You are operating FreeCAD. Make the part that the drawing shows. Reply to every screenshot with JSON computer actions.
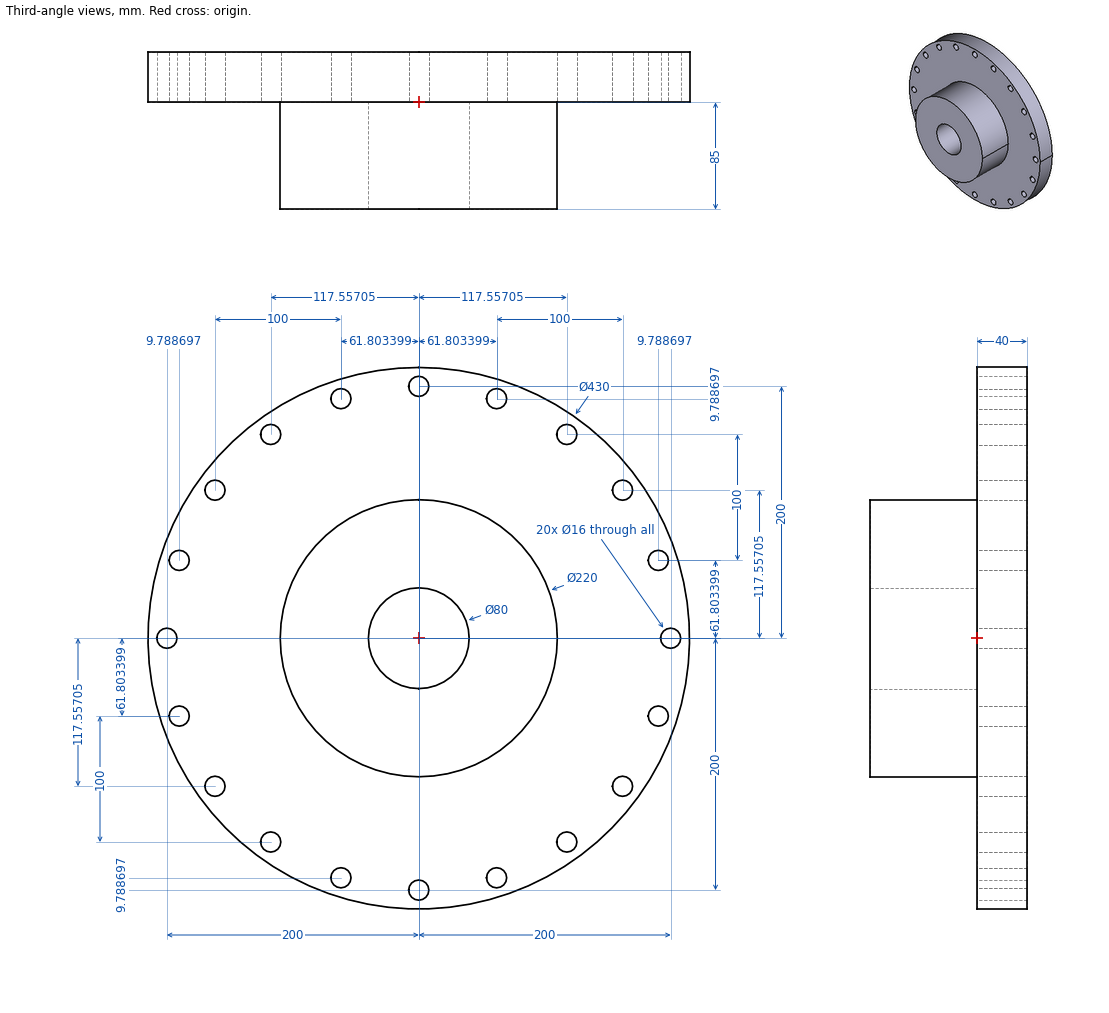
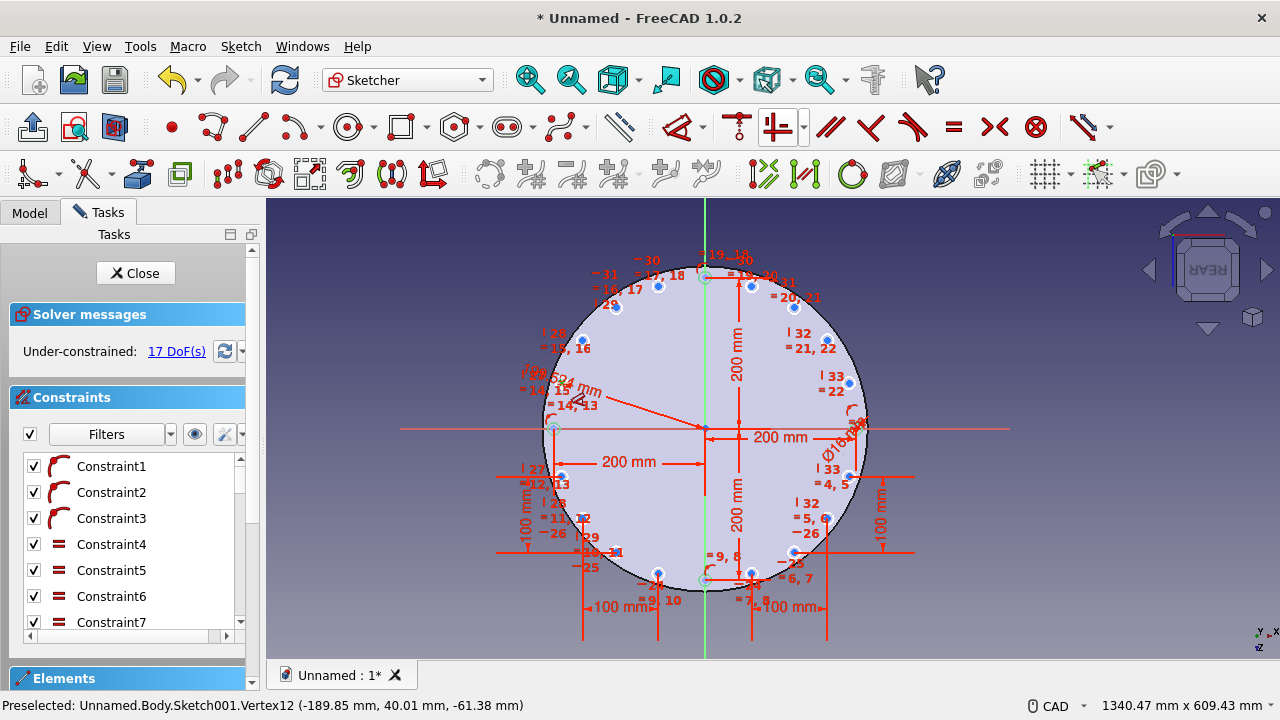
{"action": "left_click", "coordinate": [616, 308]}
{"action": "left_click", "coordinate": [528, 345]}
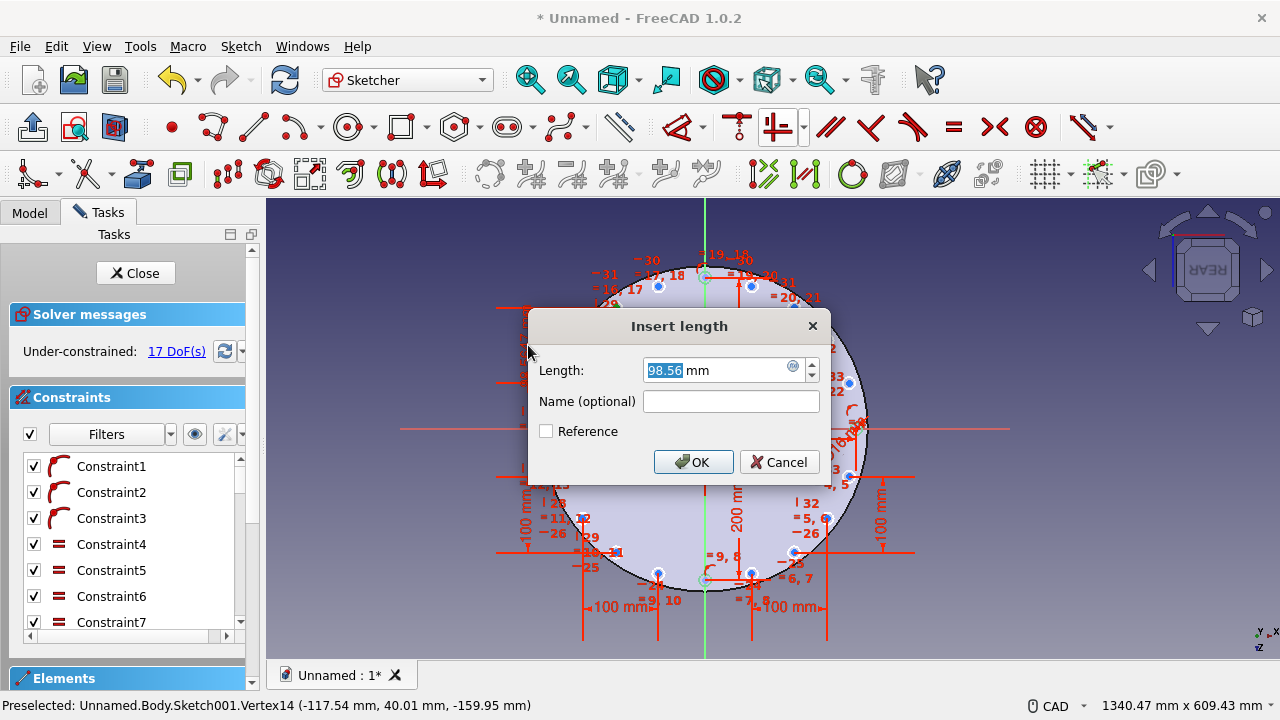
{"action": "type", "text": "100"}
{"action": "key", "text": "Return"}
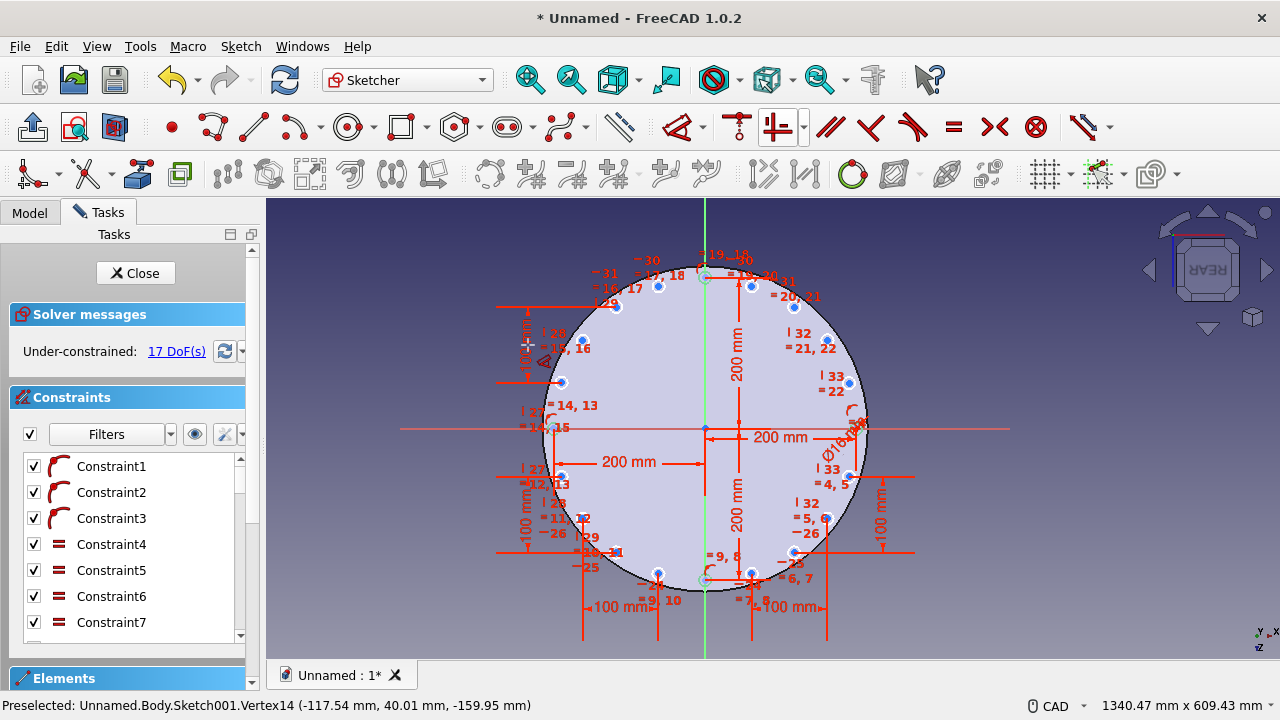
{"action": "left_click", "coordinate": [583, 341]}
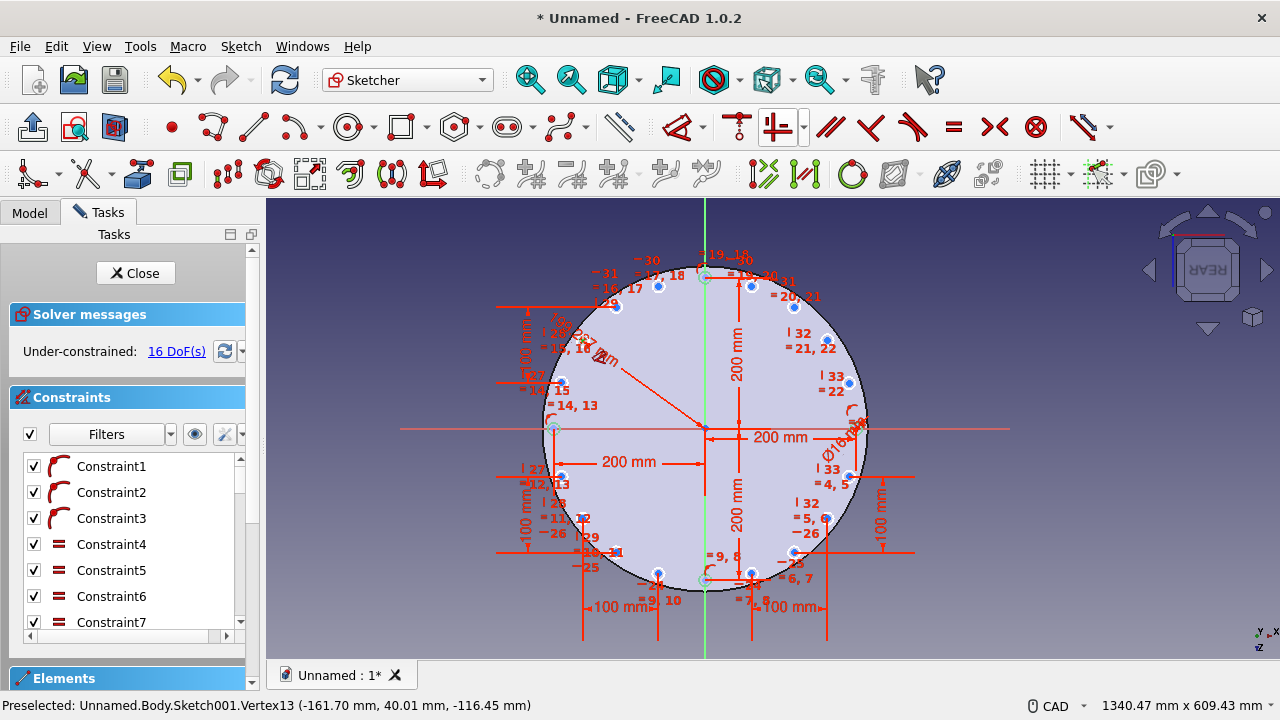
{"action": "left_click", "coordinate": [659, 286]}
{"action": "left_click", "coordinate": [621, 252]}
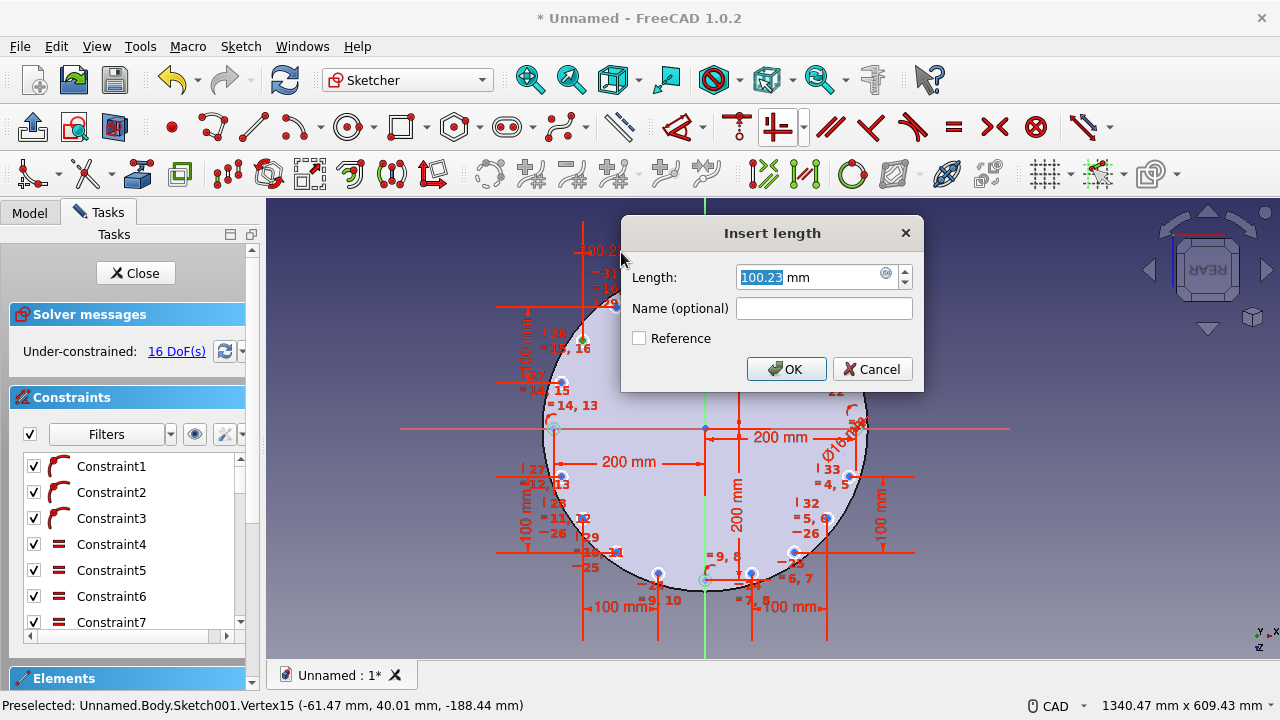
{"action": "type", "text": "100"}
{"action": "key", "text": "Return"}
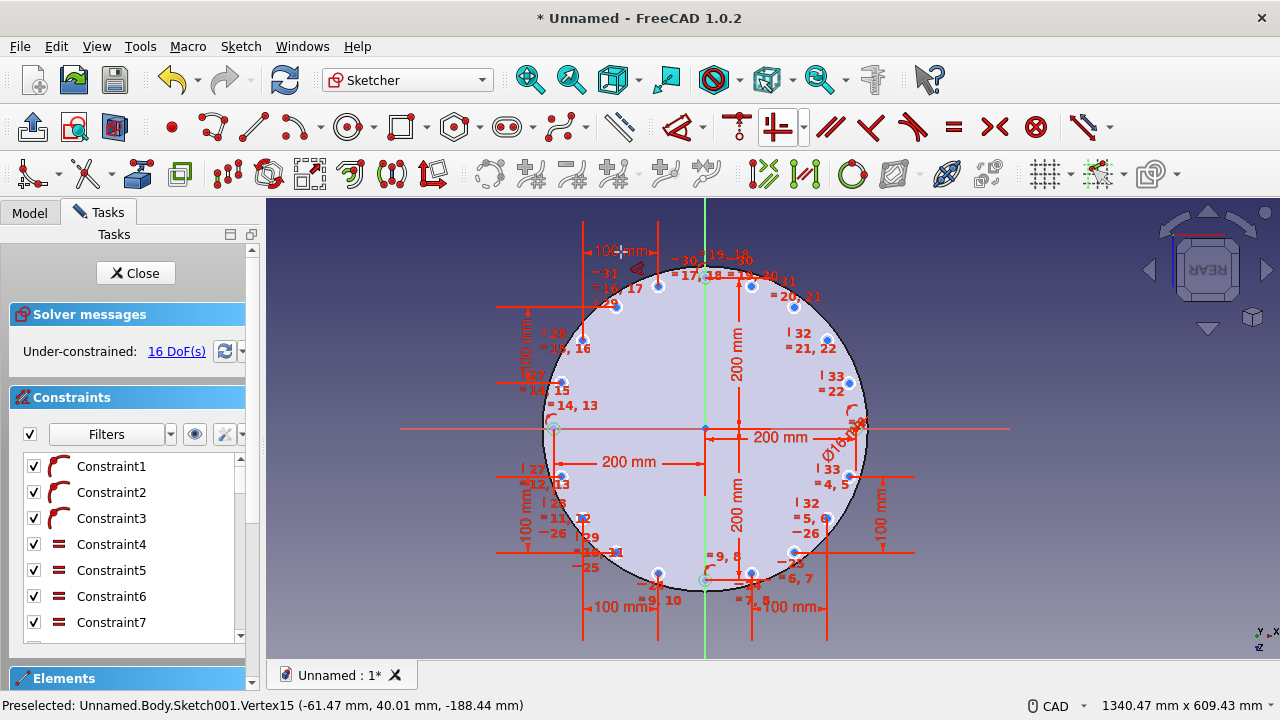
{"action": "left_click", "coordinate": [752, 286]}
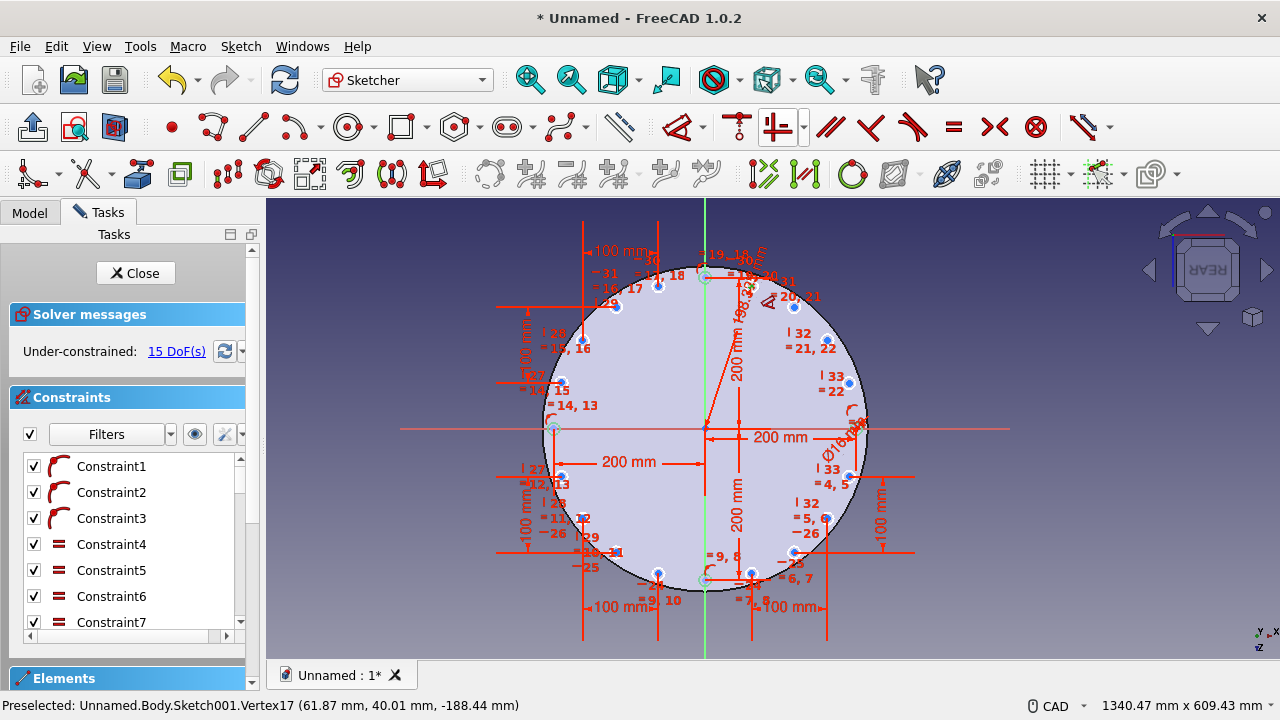
{"action": "left_click", "coordinate": [827, 340]}
{"action": "left_click", "coordinate": [790, 252]}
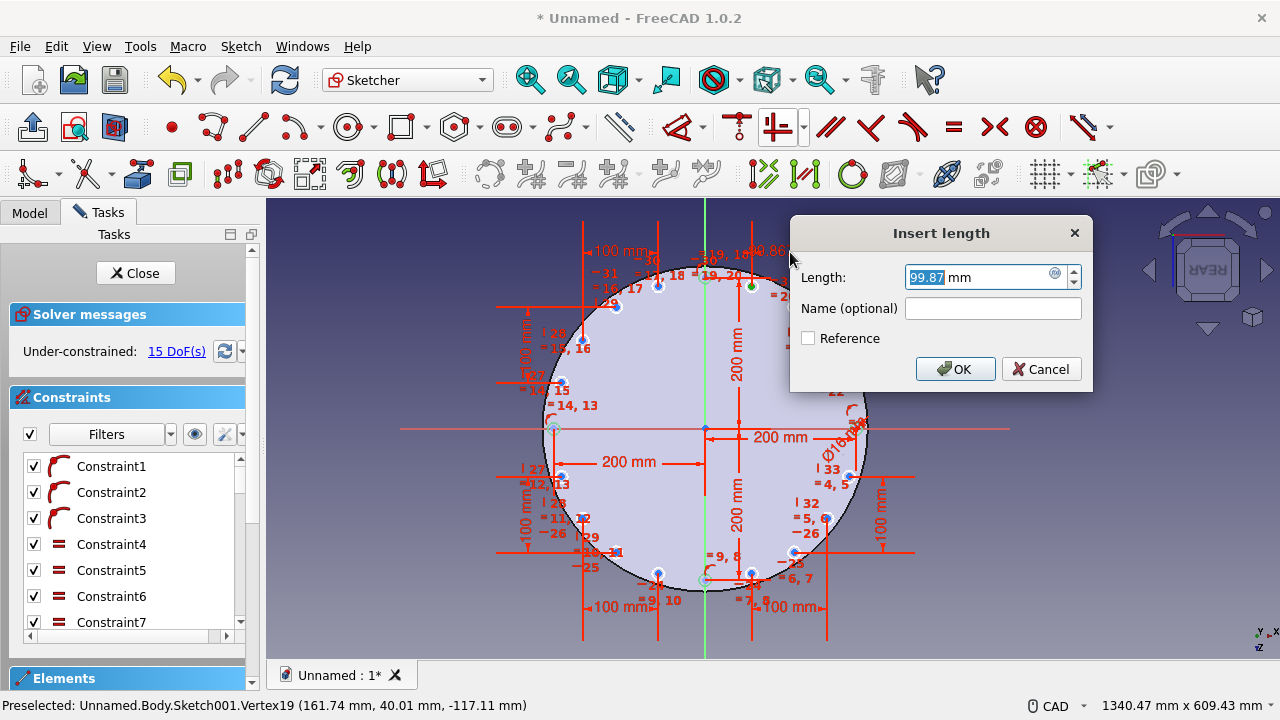
{"action": "type", "text": "100"}
{"action": "key", "text": "Return"}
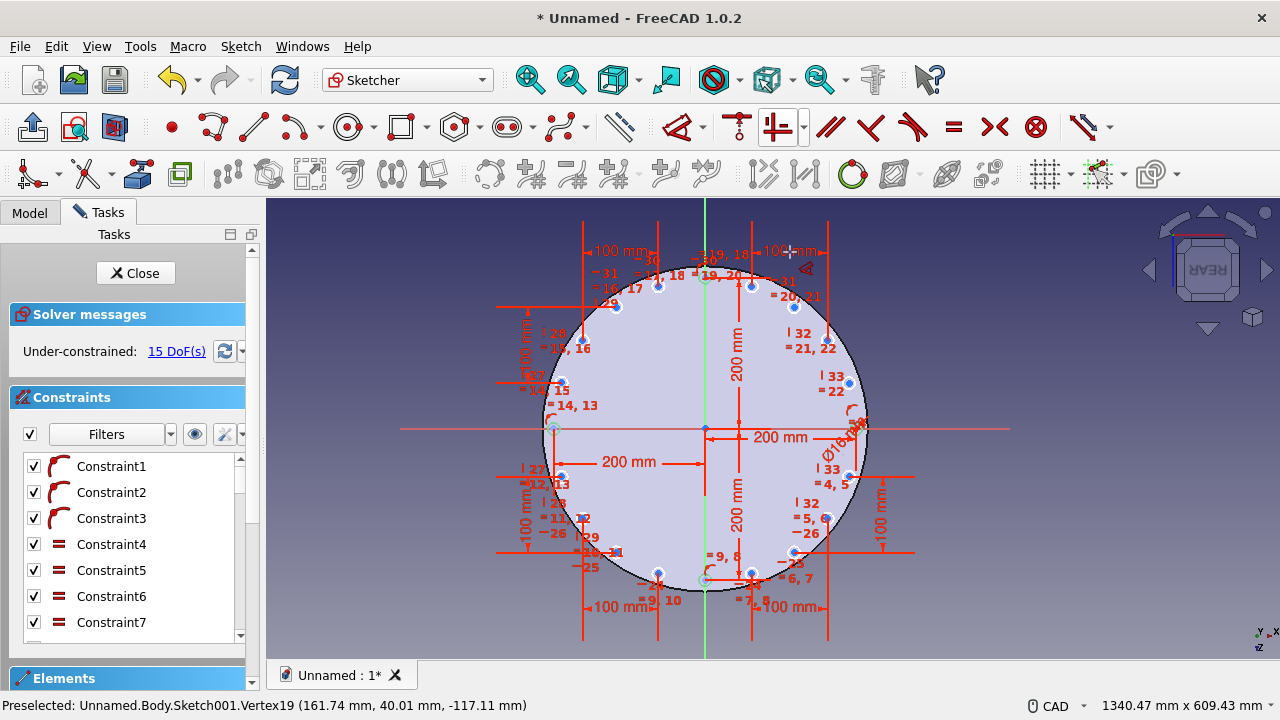
{"action": "left_click", "coordinate": [794, 307]}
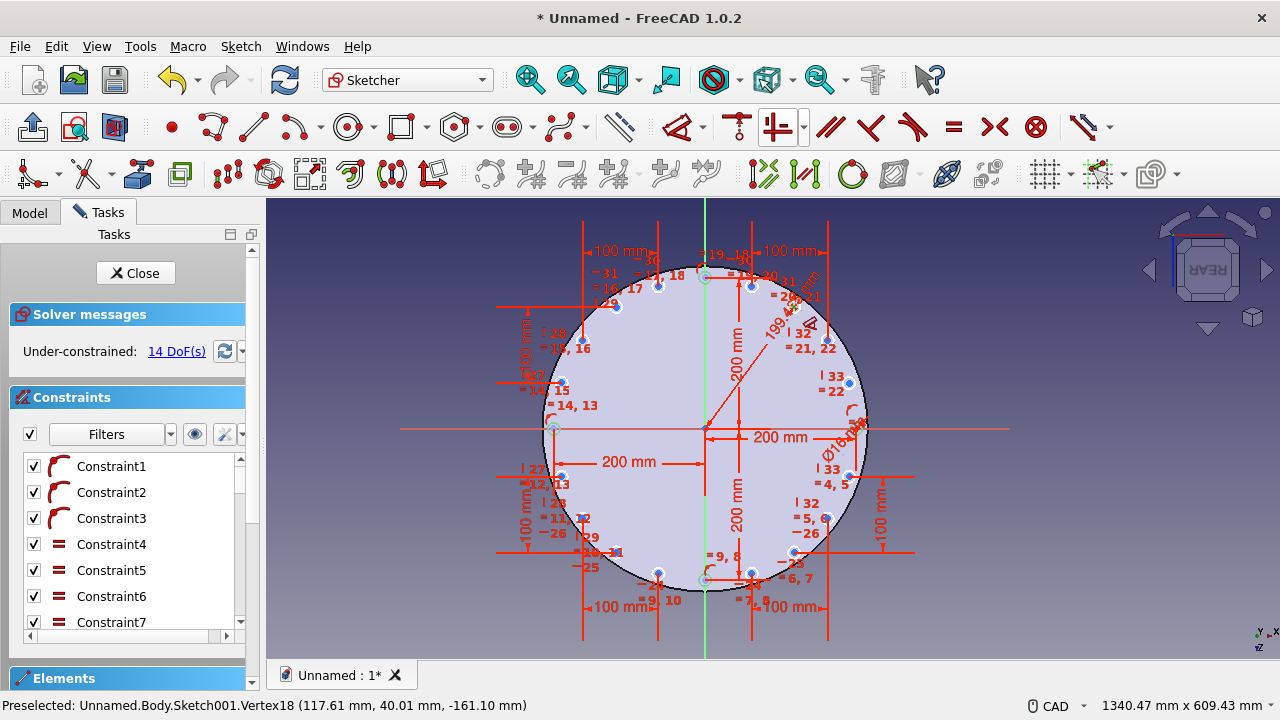
{"action": "left_click", "coordinate": [849, 383]}
{"action": "left_click", "coordinate": [883, 345]}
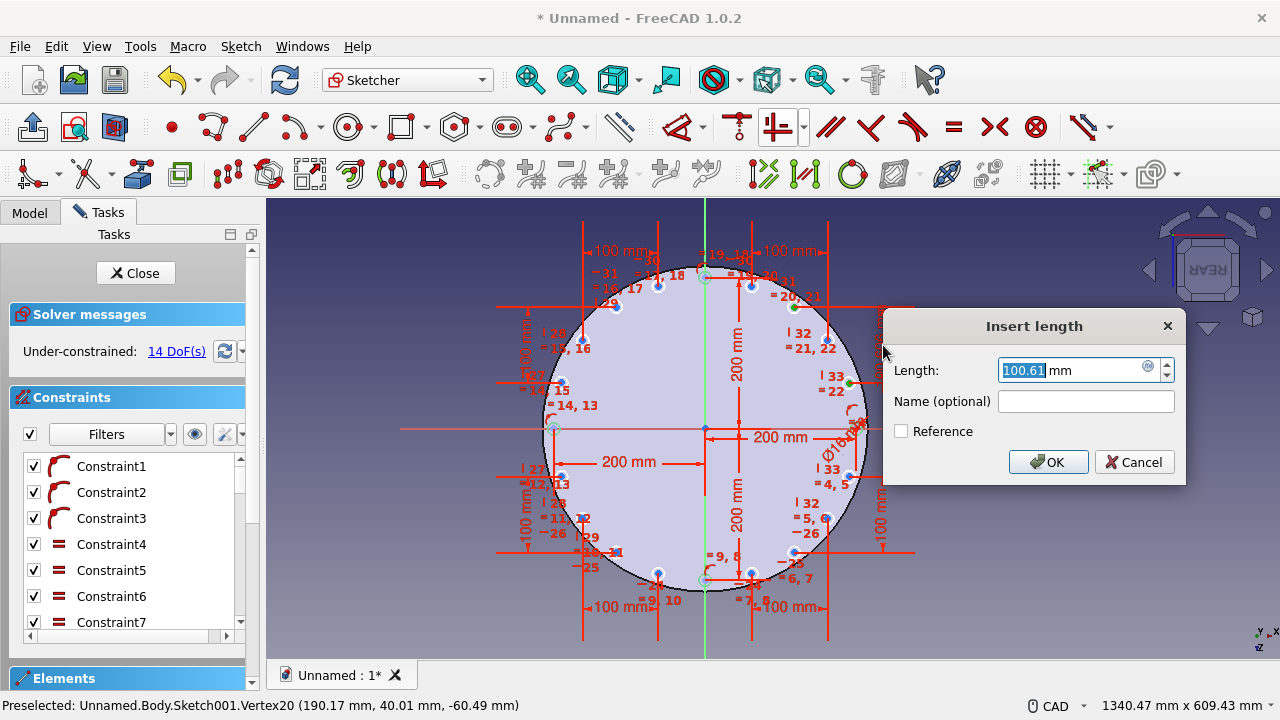
{"action": "type", "text": "100"}
{"action": "key", "text": "Return"}